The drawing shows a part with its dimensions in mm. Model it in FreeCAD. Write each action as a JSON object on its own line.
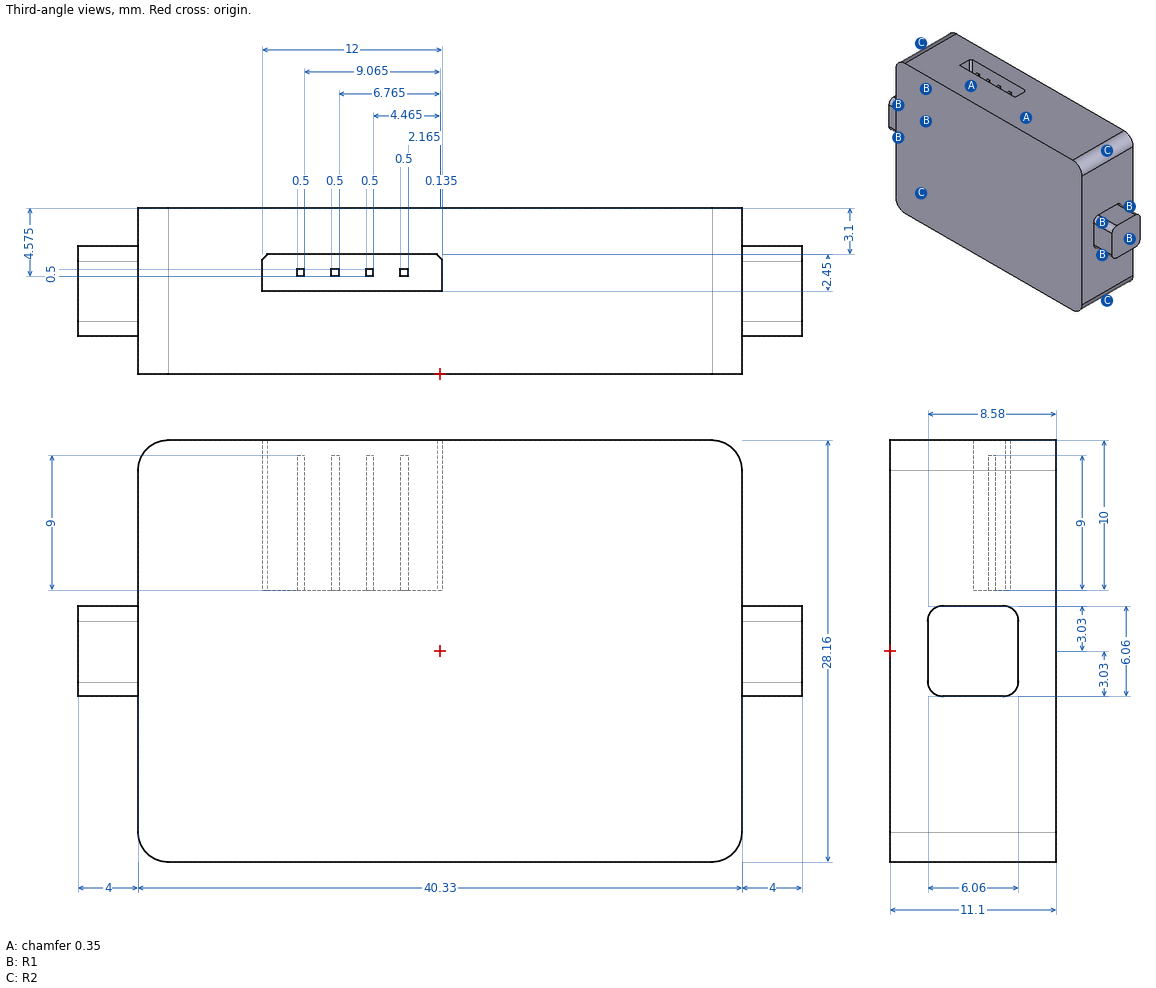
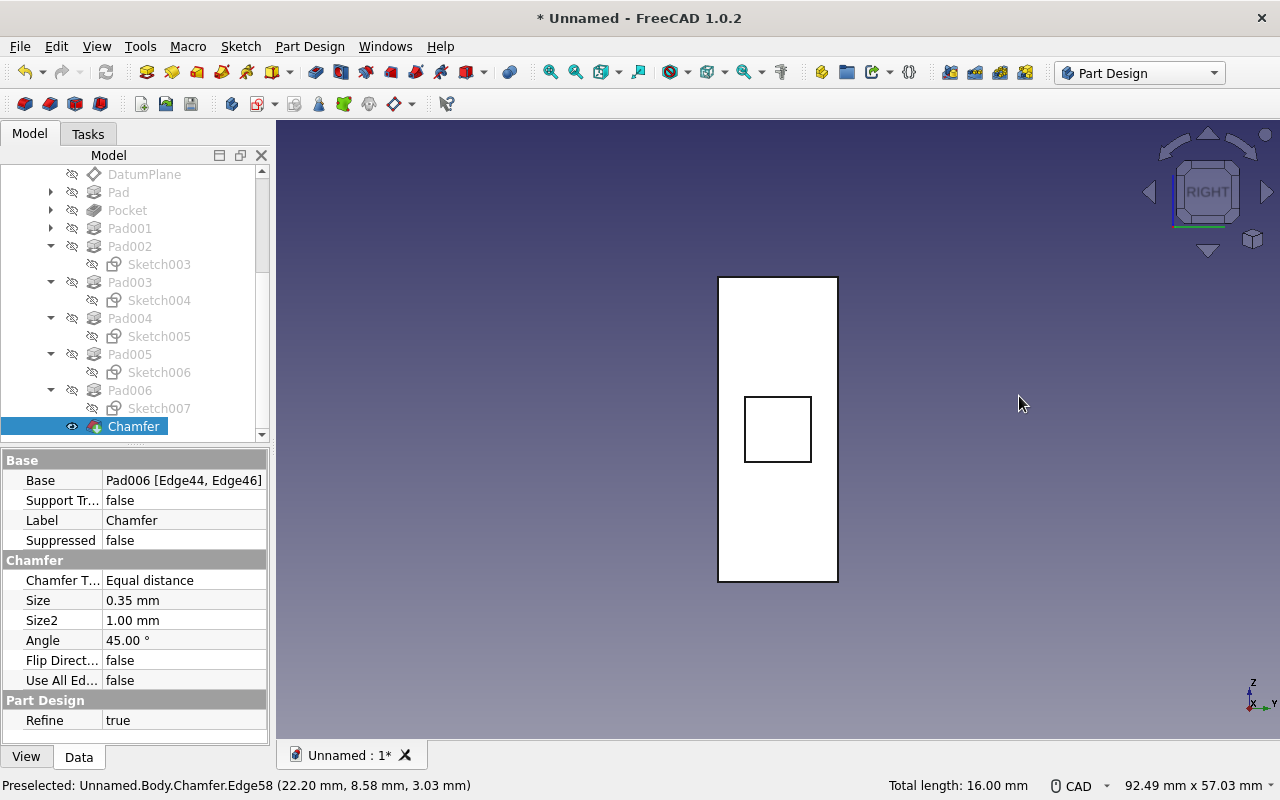
{"action": "key", "text": "5"}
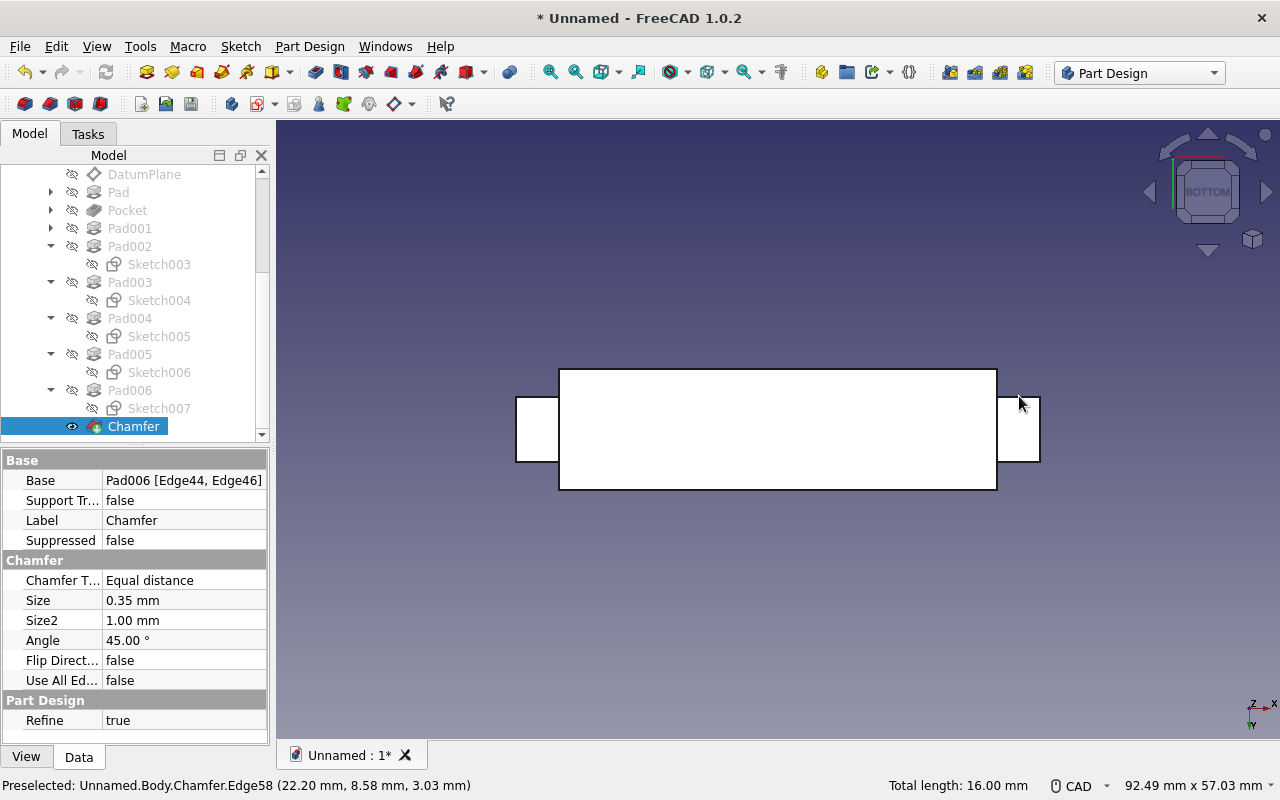
{"action": "left_click", "coordinate": [537, 396], "text": "ctrl"}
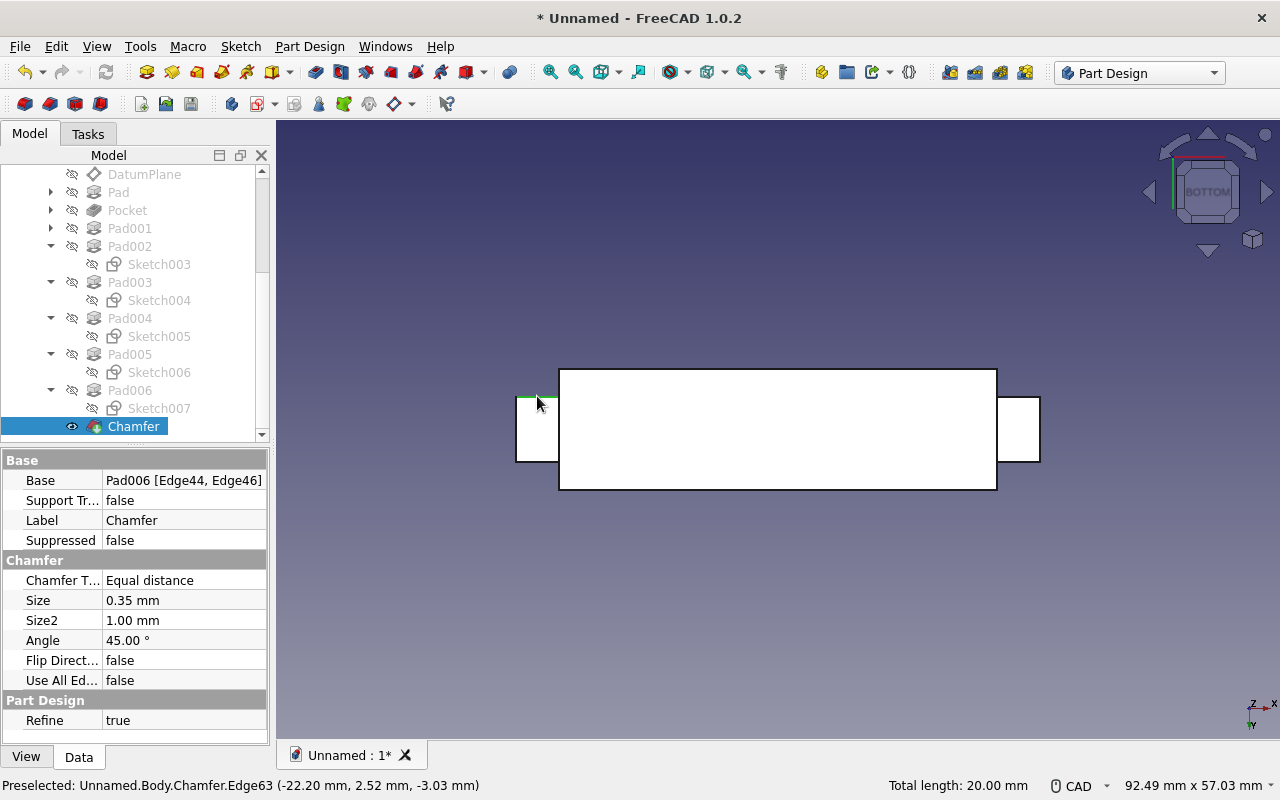
{"action": "left_click", "coordinate": [1019, 396], "text": "ctrl"}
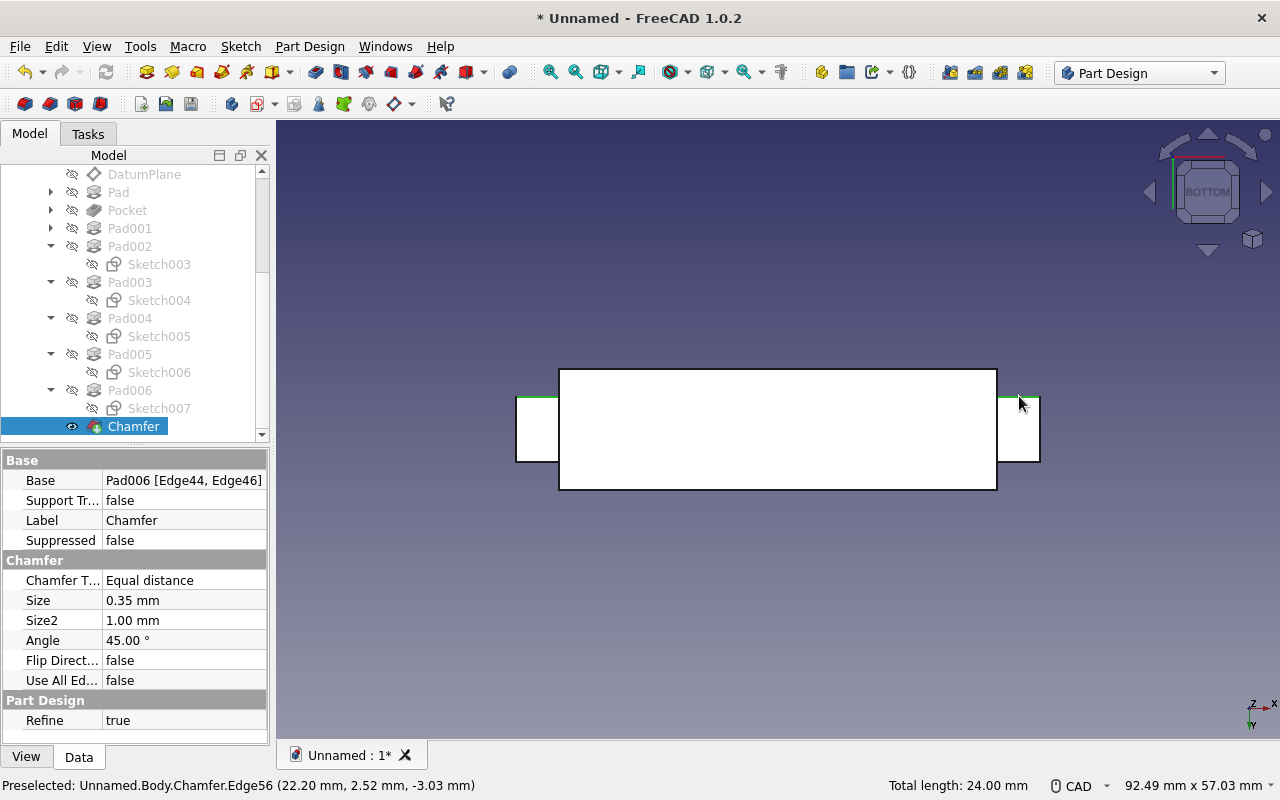
{"action": "key", "text": "4"}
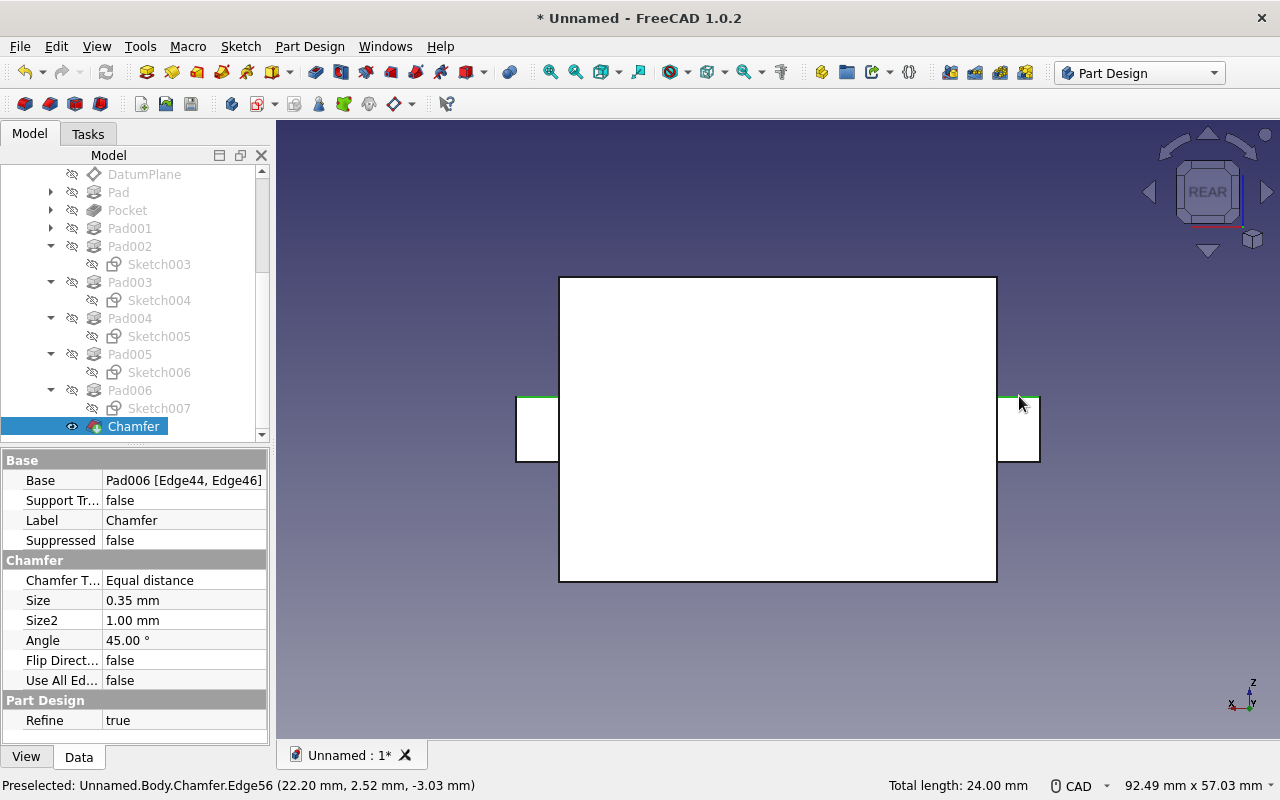
{"action": "left_click", "coordinate": [1019, 461], "text": "ctrl"}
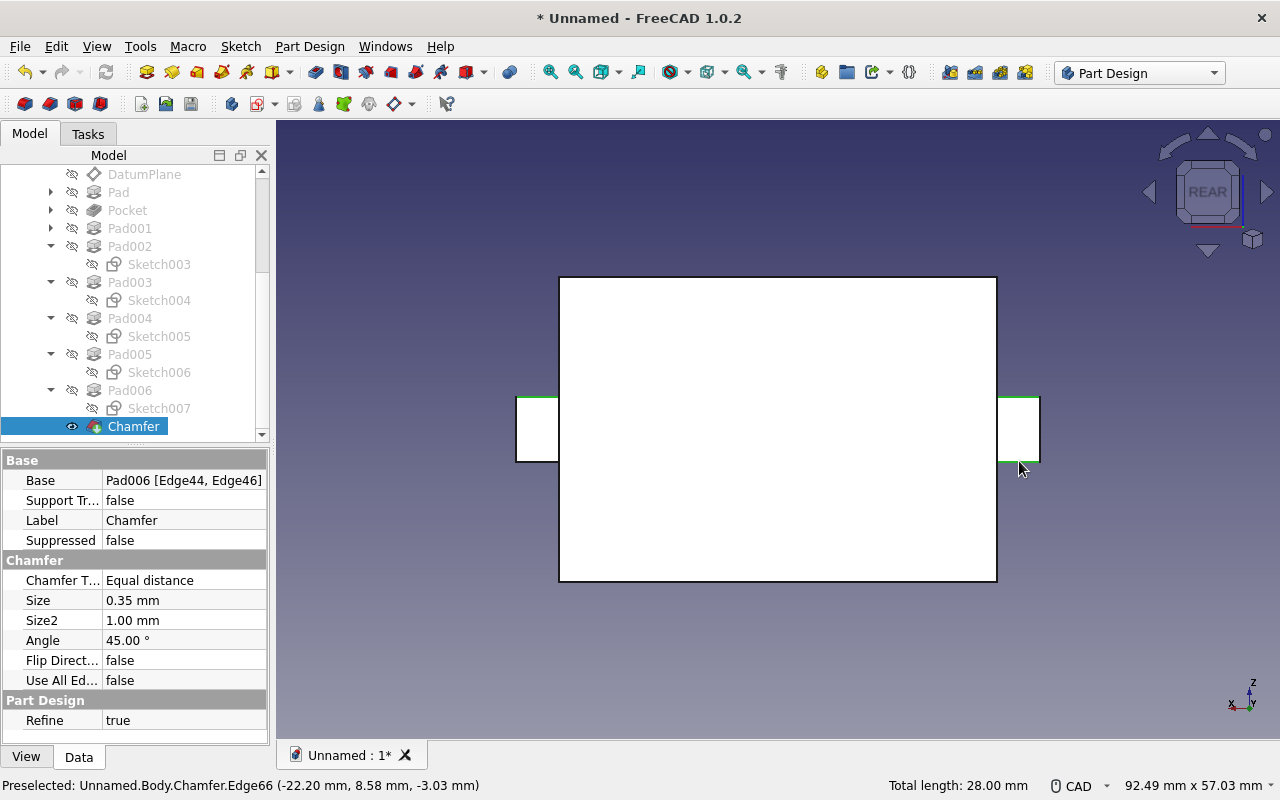
{"action": "left_click", "coordinate": [537, 461], "text": "ctrl"}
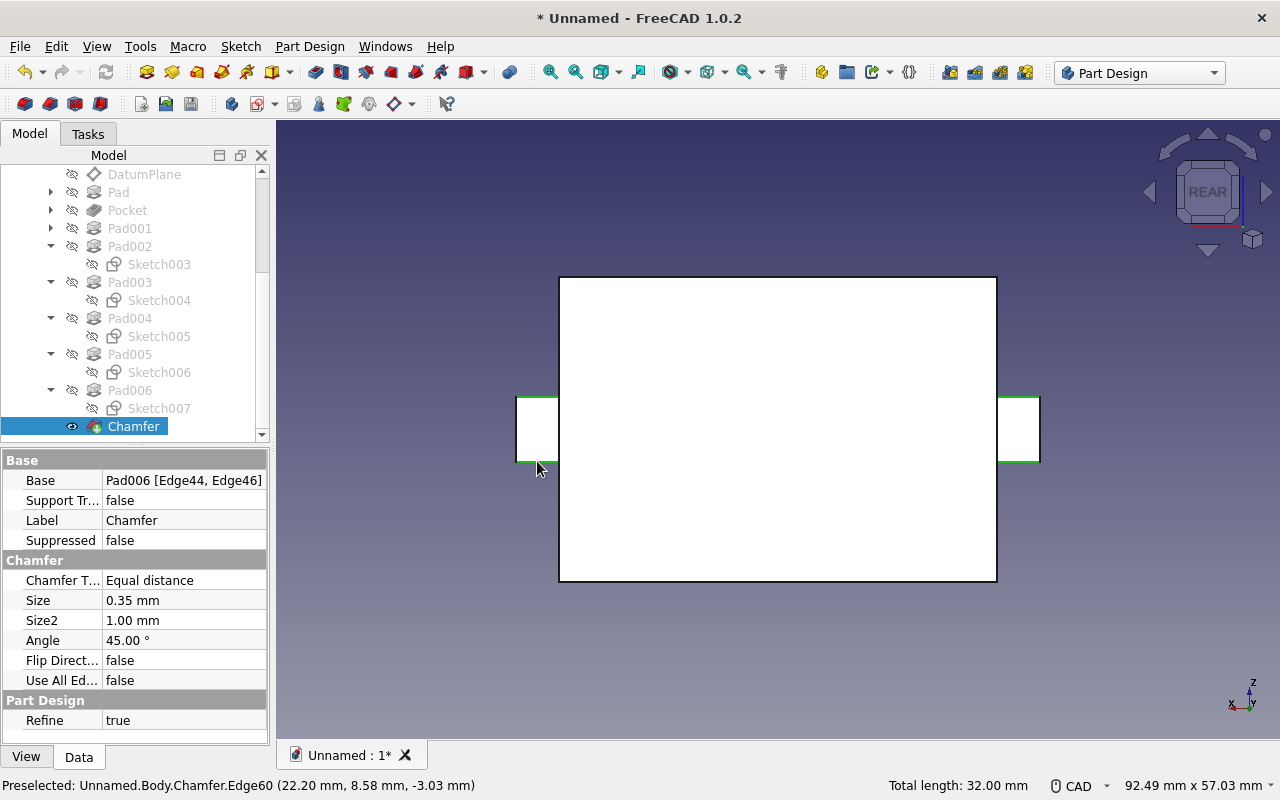
{"action": "left_click", "coordinate": [25, 104]}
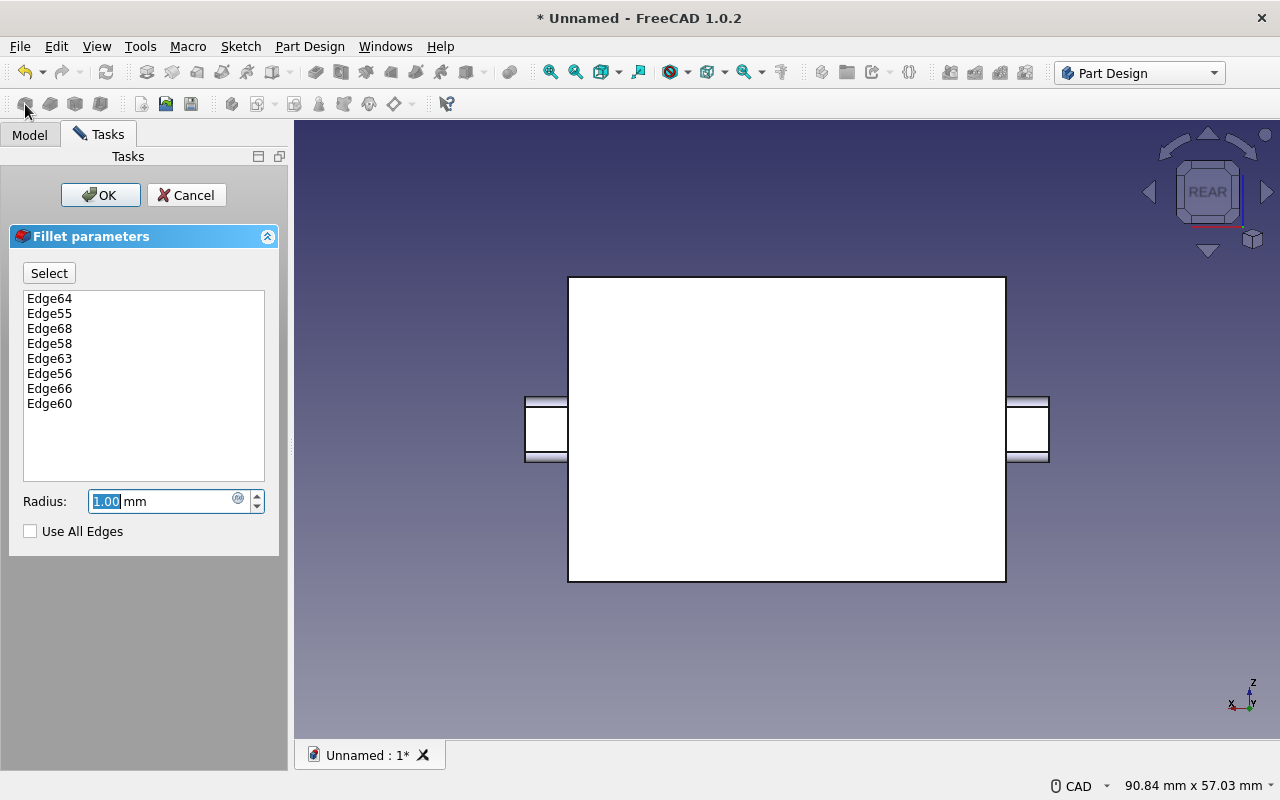
{"action": "type", "text": "1"}
{"action": "key", "text": "Tab"}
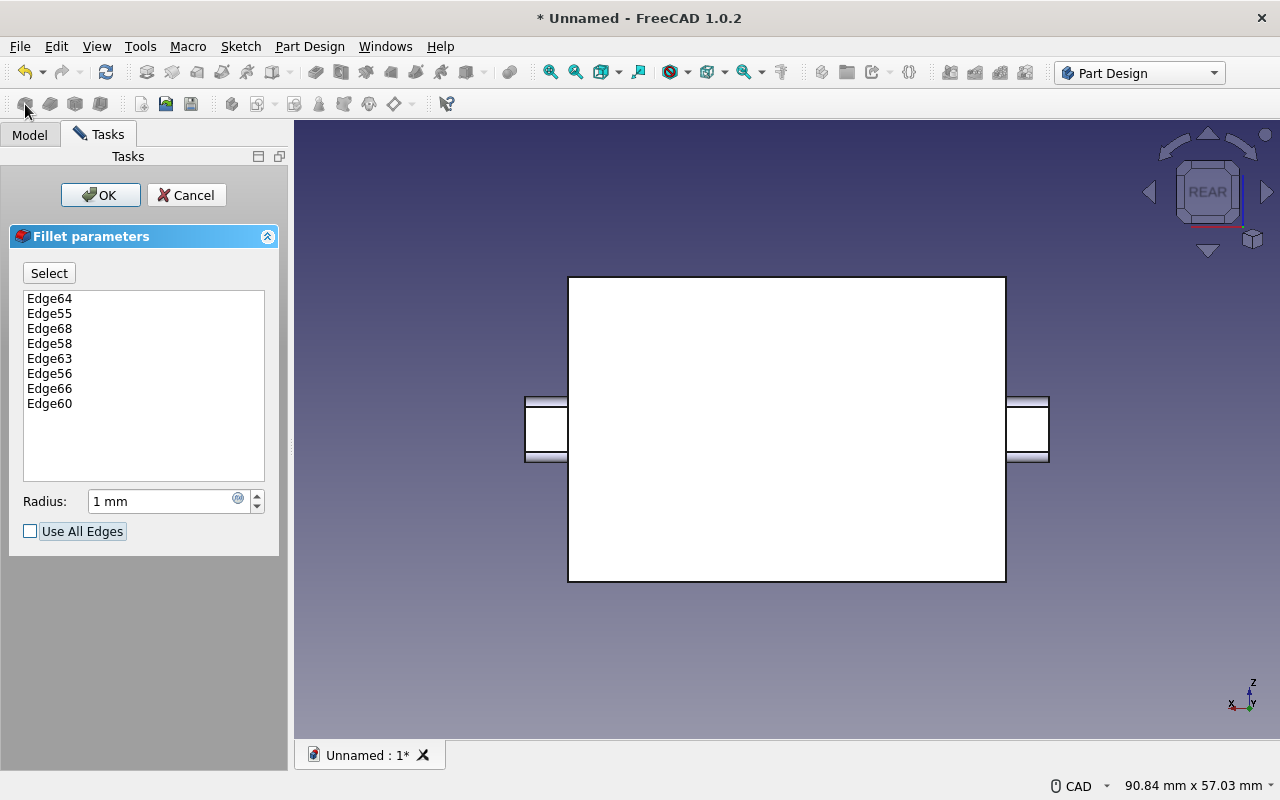
{"action": "left_click", "coordinate": [101, 195]}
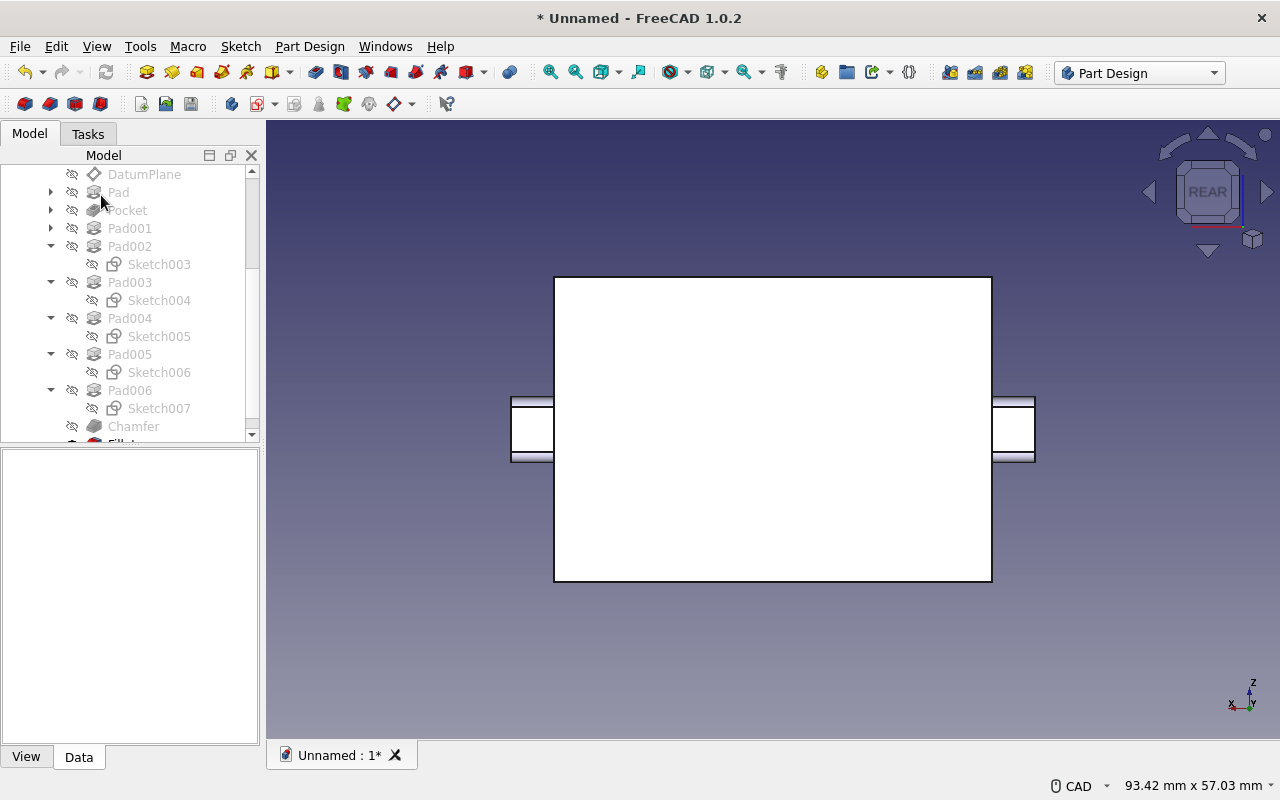
{"action": "key", "text": "0"}